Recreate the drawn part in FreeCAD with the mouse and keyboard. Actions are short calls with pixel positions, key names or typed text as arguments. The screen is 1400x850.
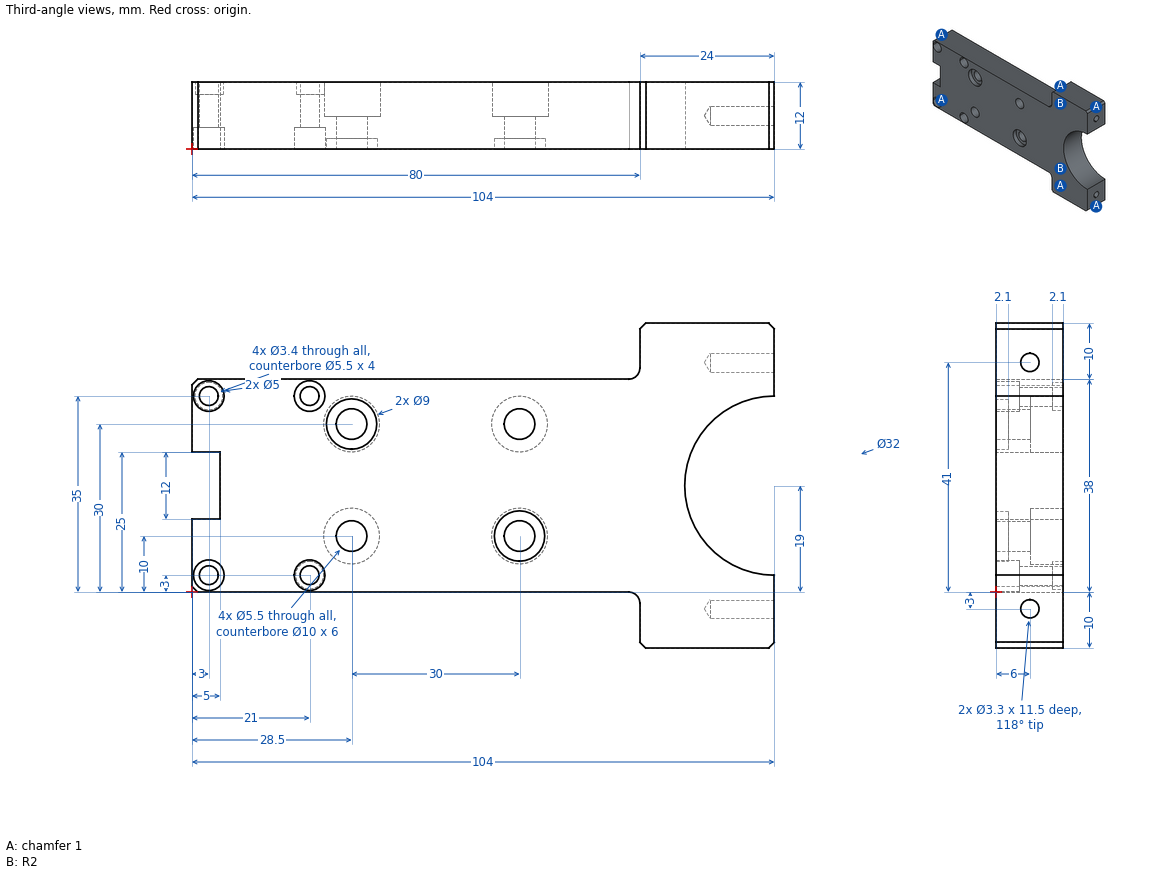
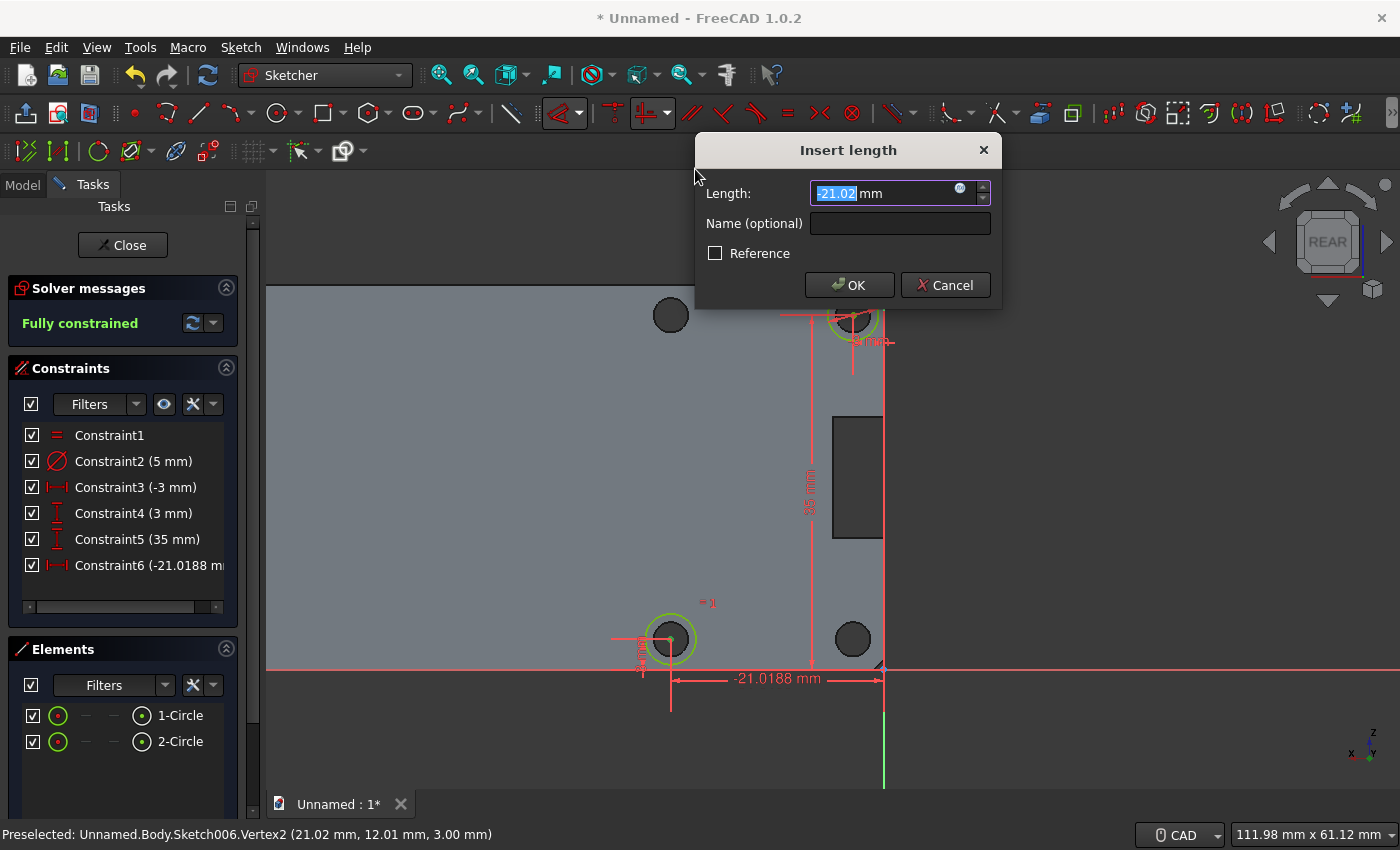
text(-21)
key(Return)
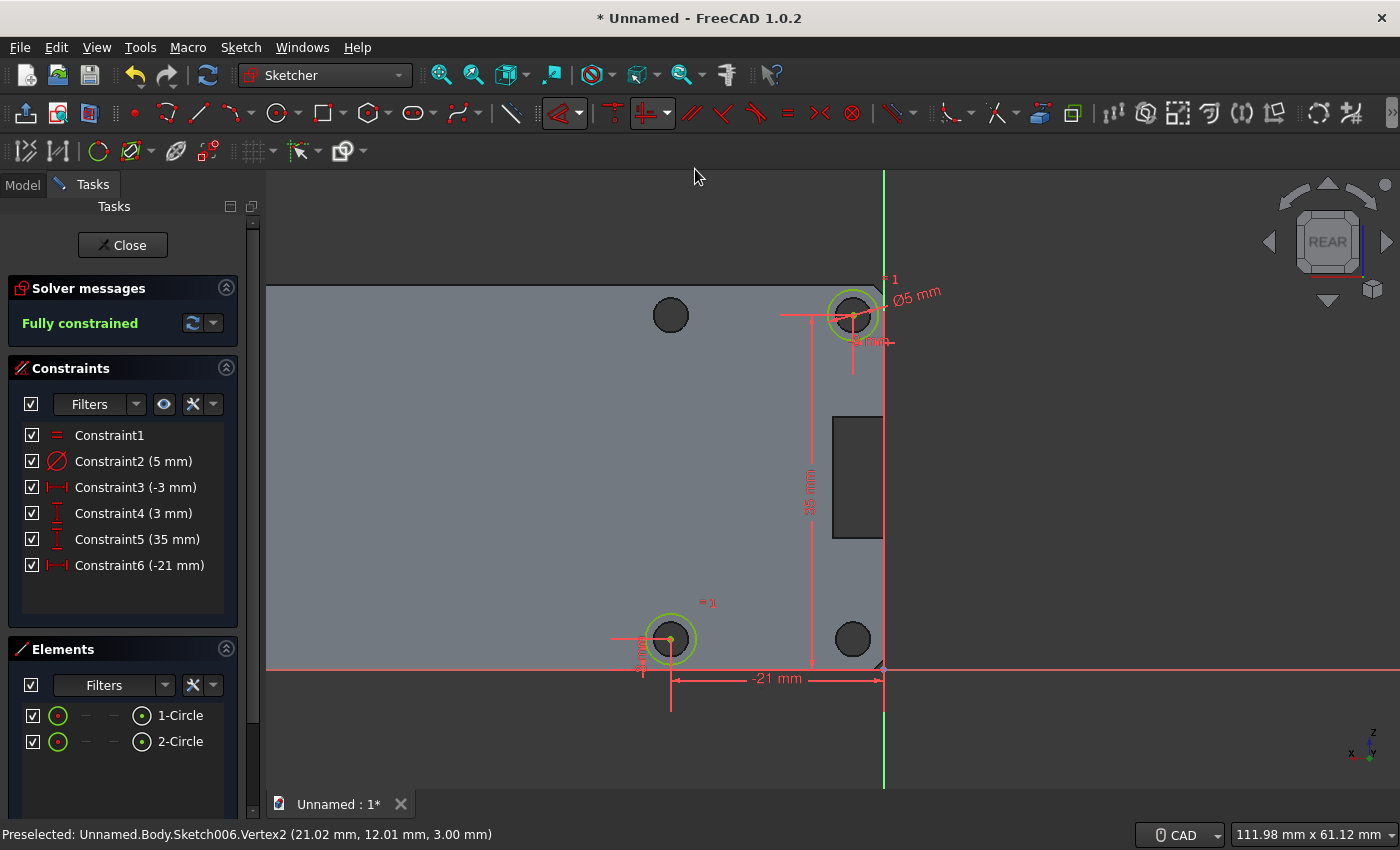
click(123, 245)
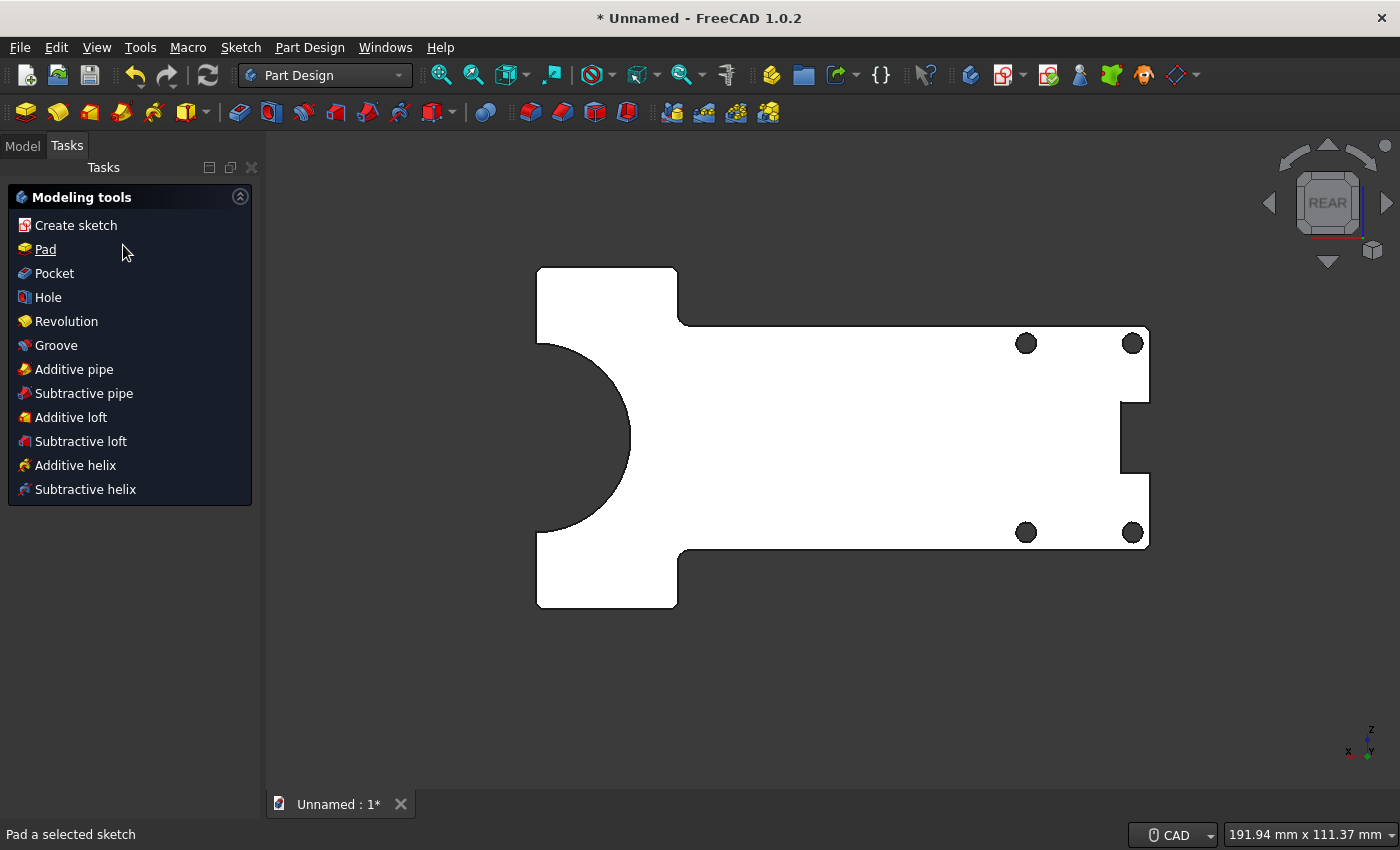
click(240, 112)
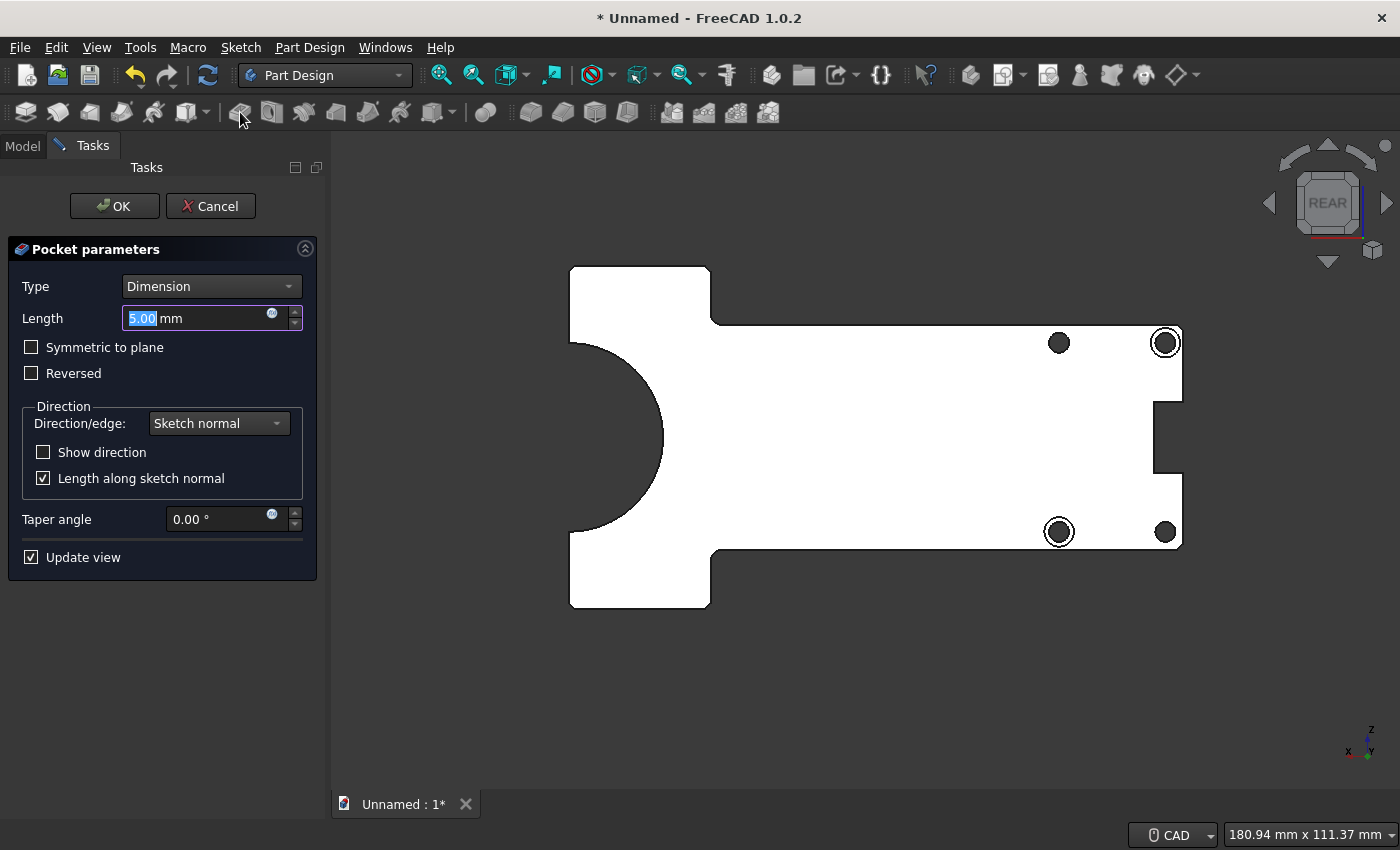
text(2.1)
key(Tab)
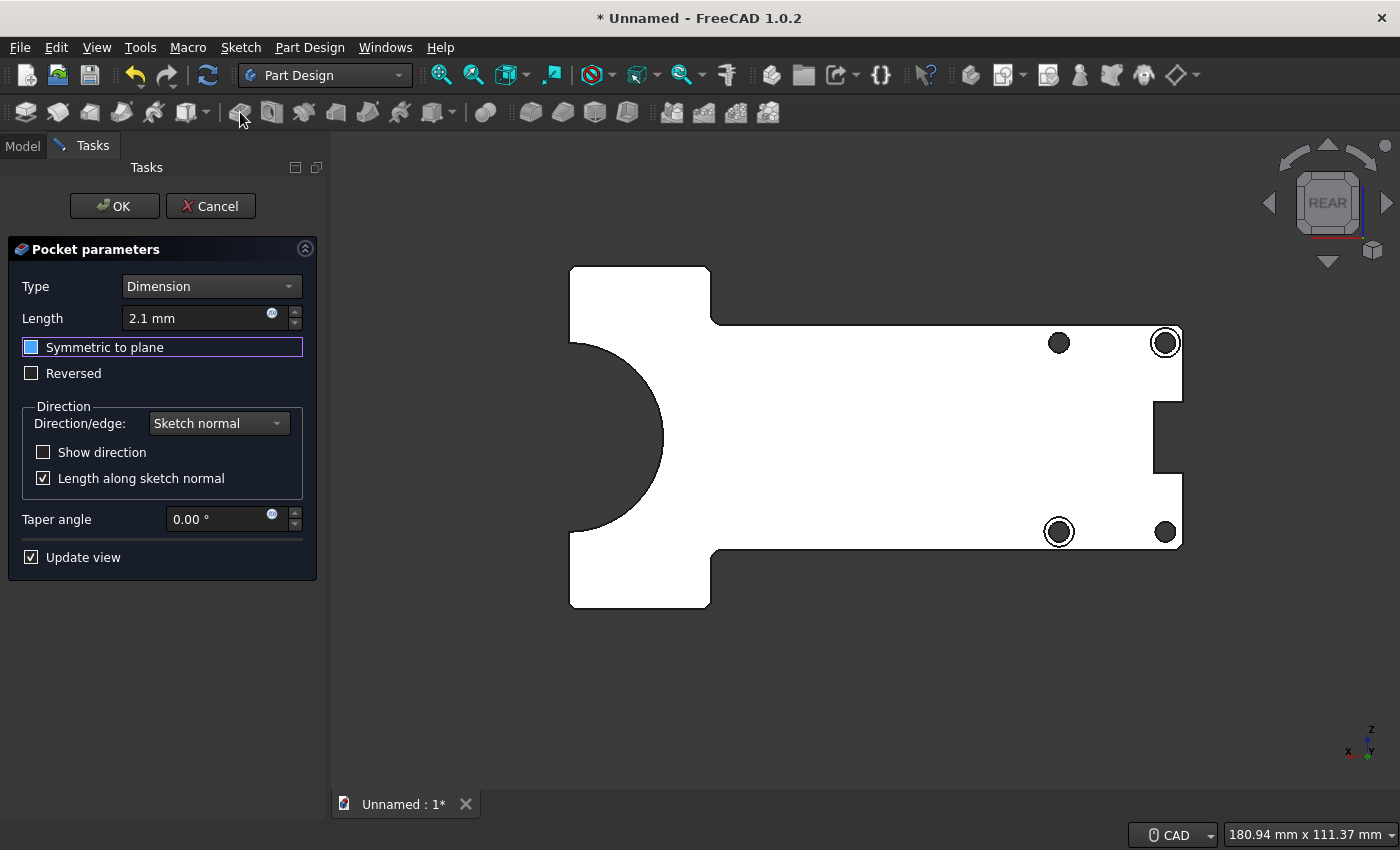
click(115, 206)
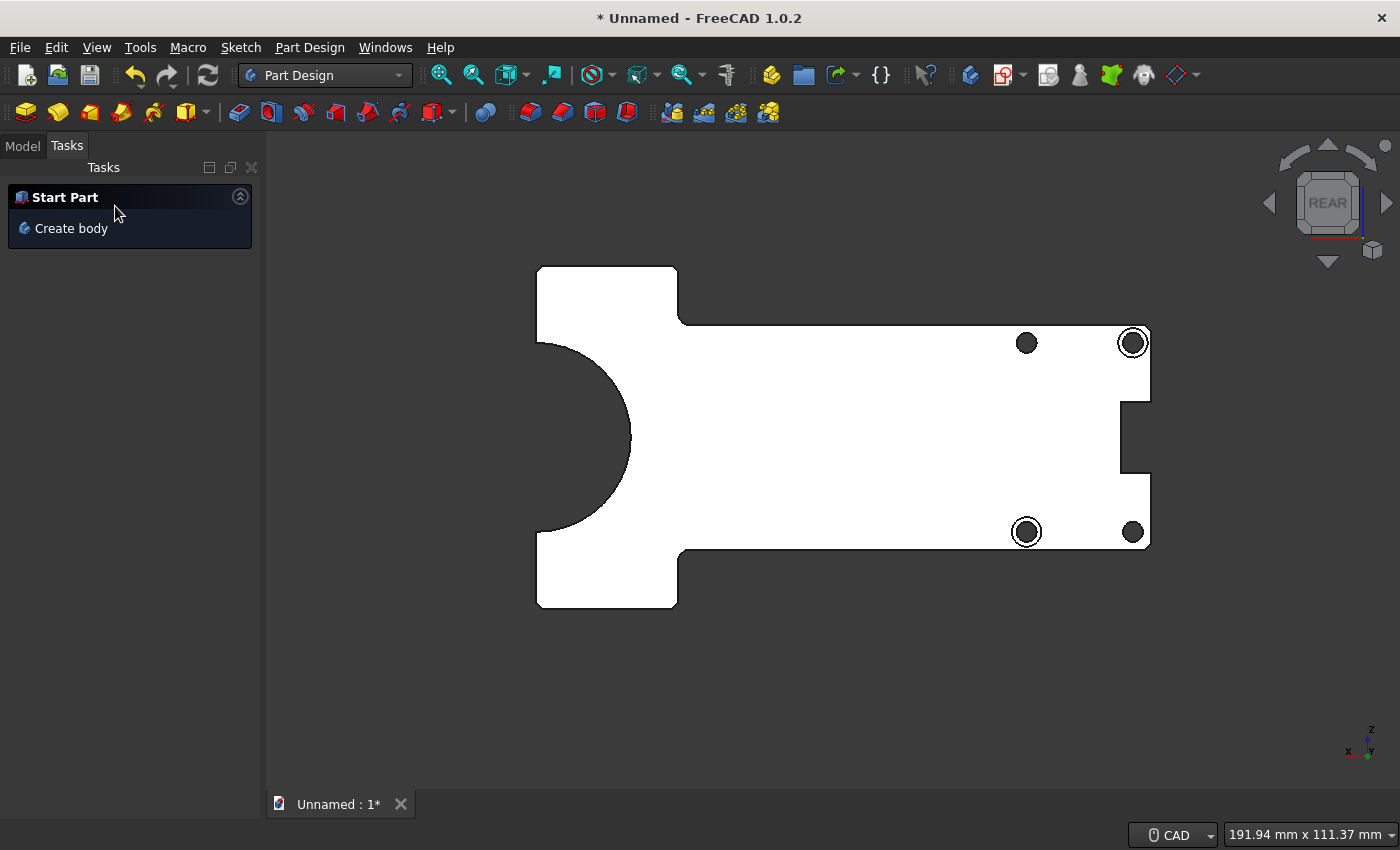
click(756, 436)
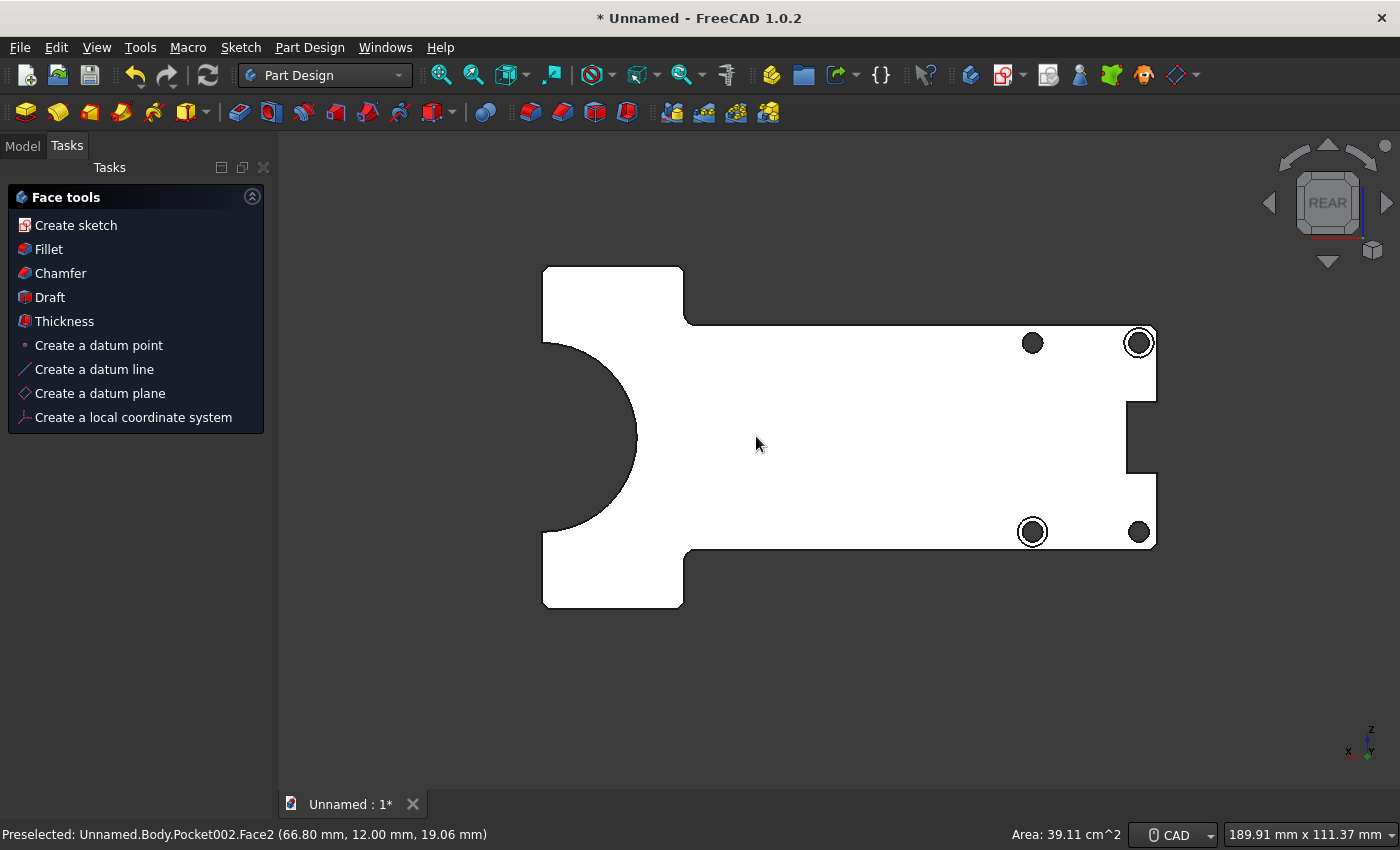
click(1004, 76)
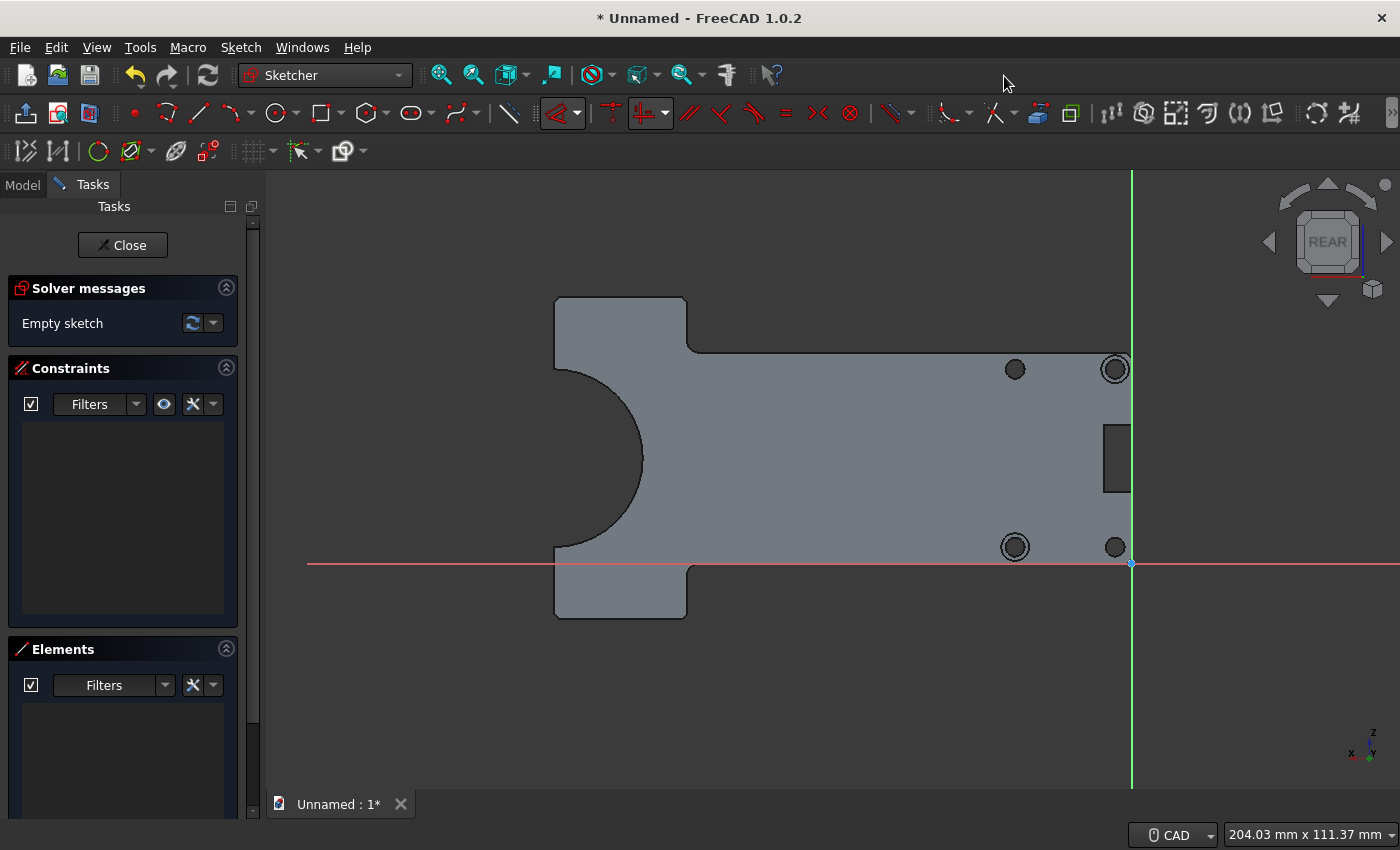
scroll(1201, 465, up, 3)